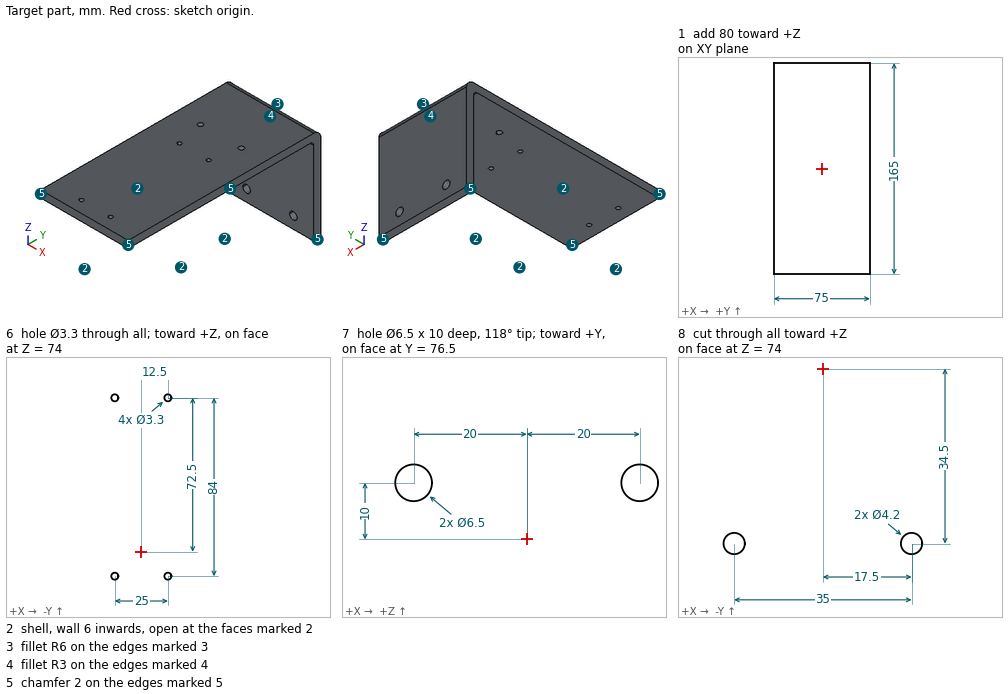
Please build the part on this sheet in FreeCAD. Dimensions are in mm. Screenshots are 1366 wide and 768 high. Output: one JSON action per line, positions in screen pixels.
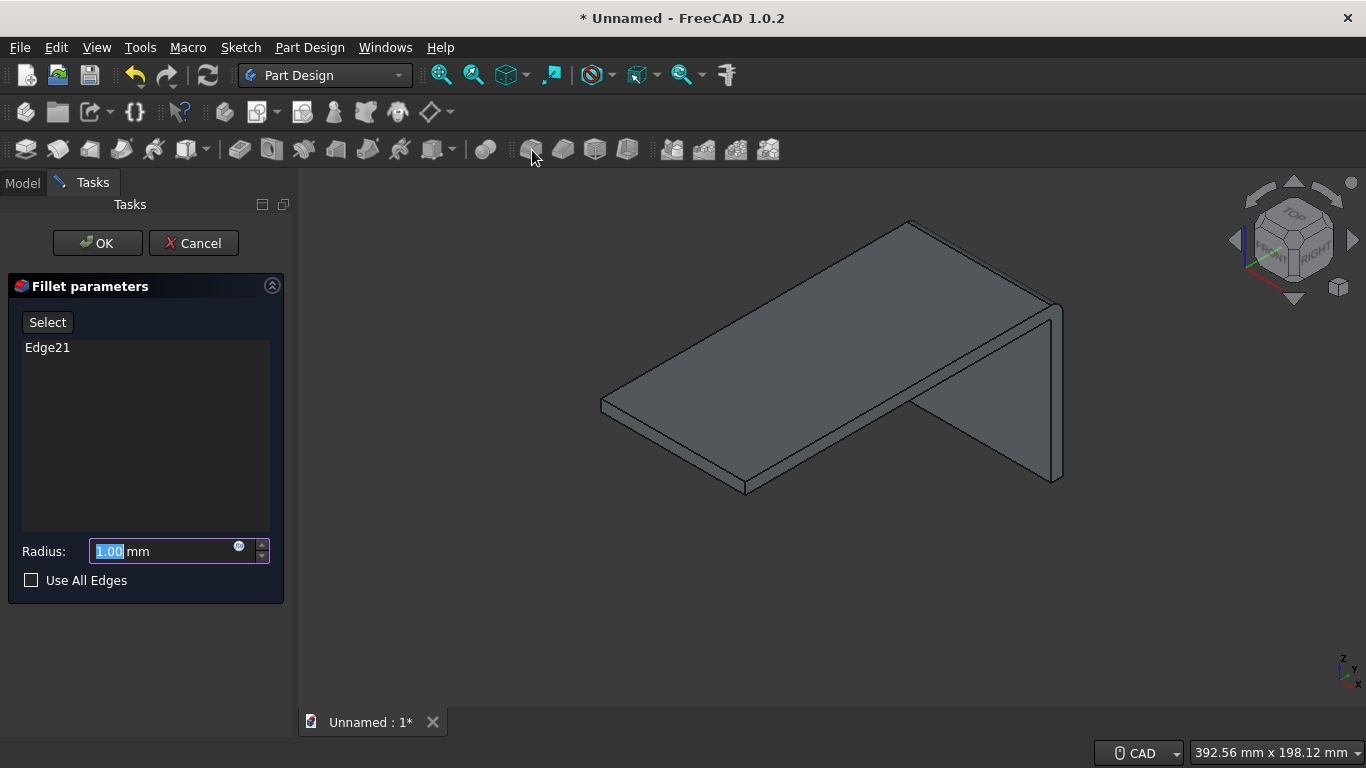
{"action": "type", "text": "3"}
{"action": "key", "text": "Tab"}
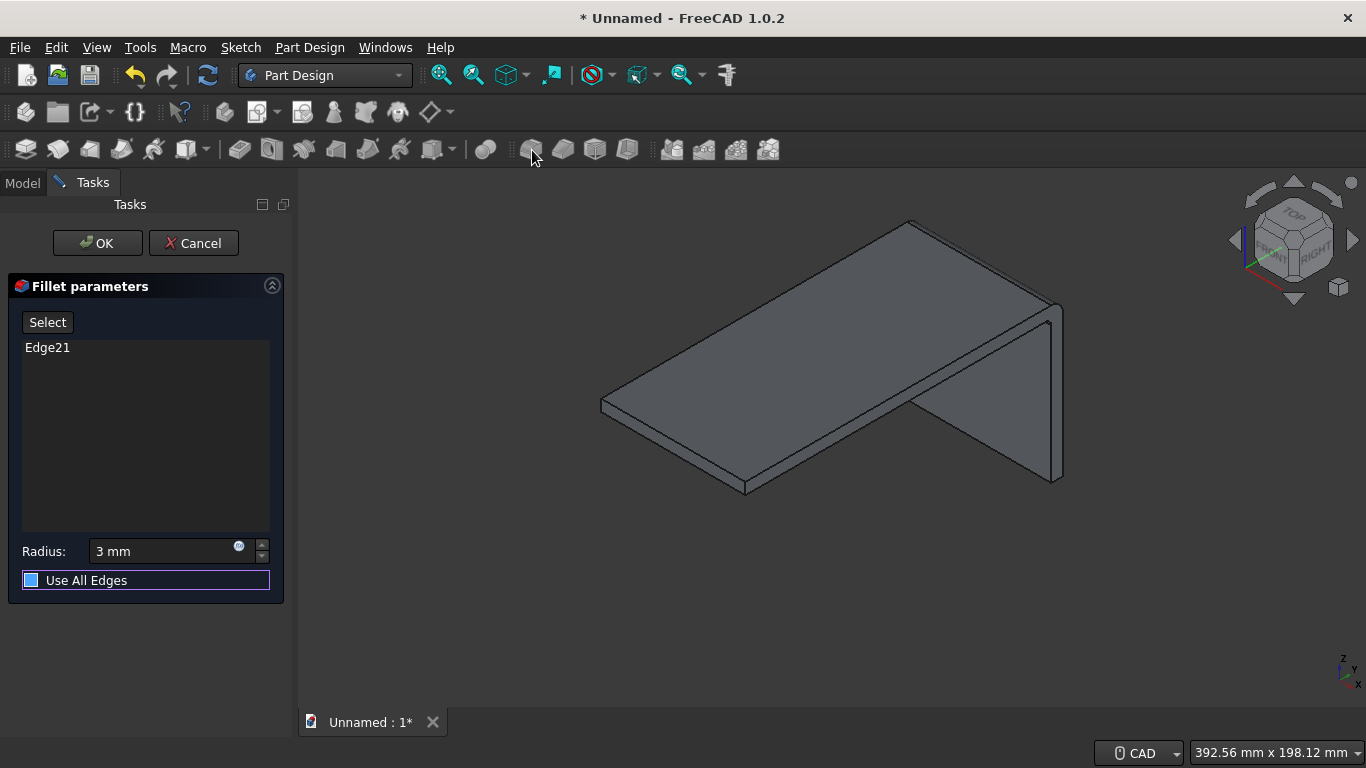
{"action": "left_click", "coordinate": [98, 243]}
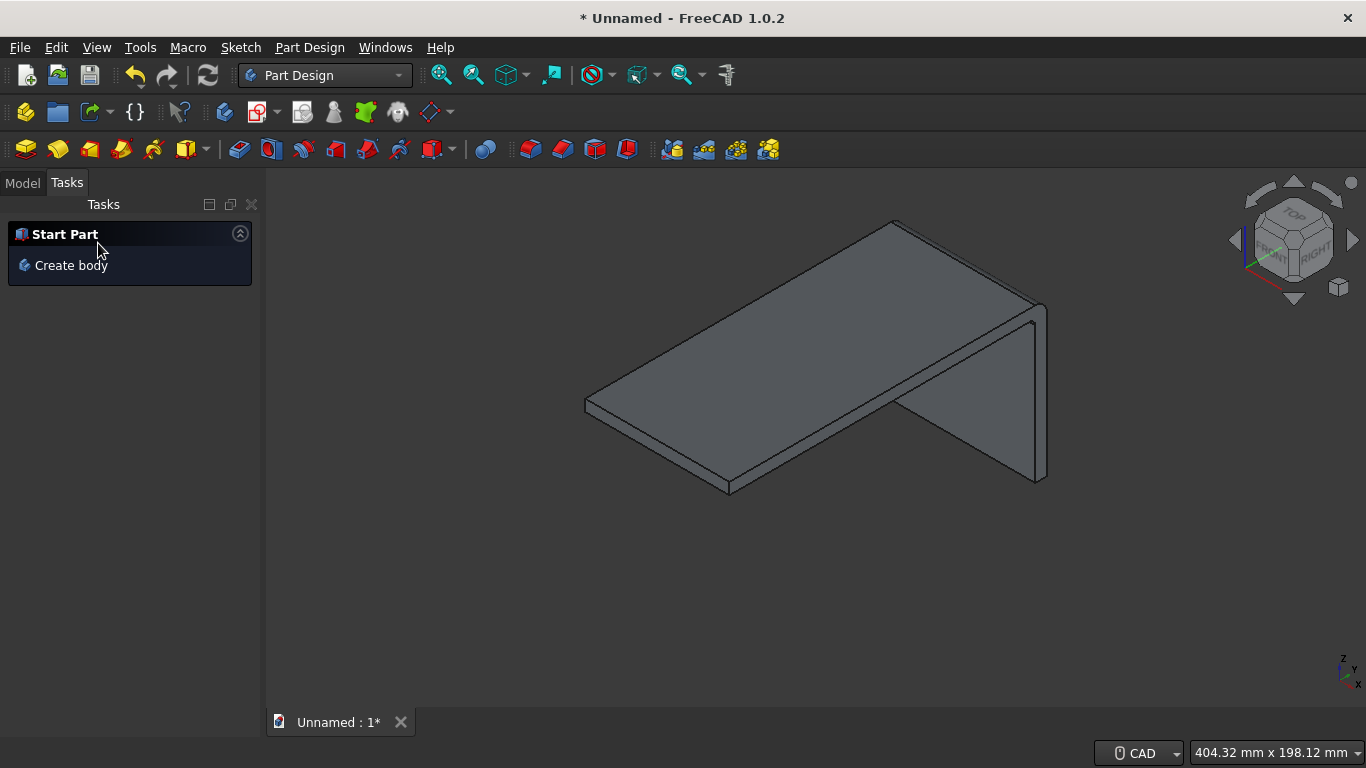
{"action": "left_click", "coordinate": [729, 488]}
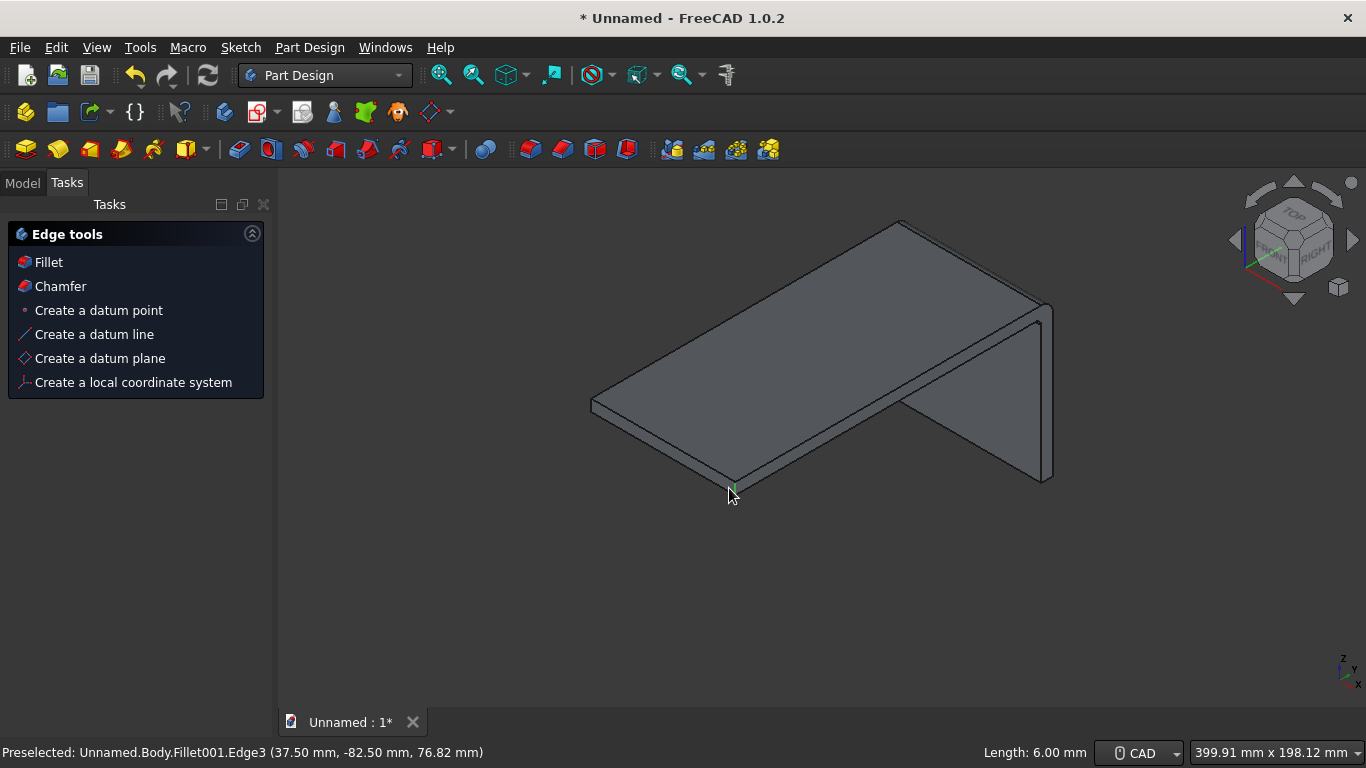
{"action": "scroll", "coordinate": [903, 395], "scroll_direction": "up", "scroll_amount": 5}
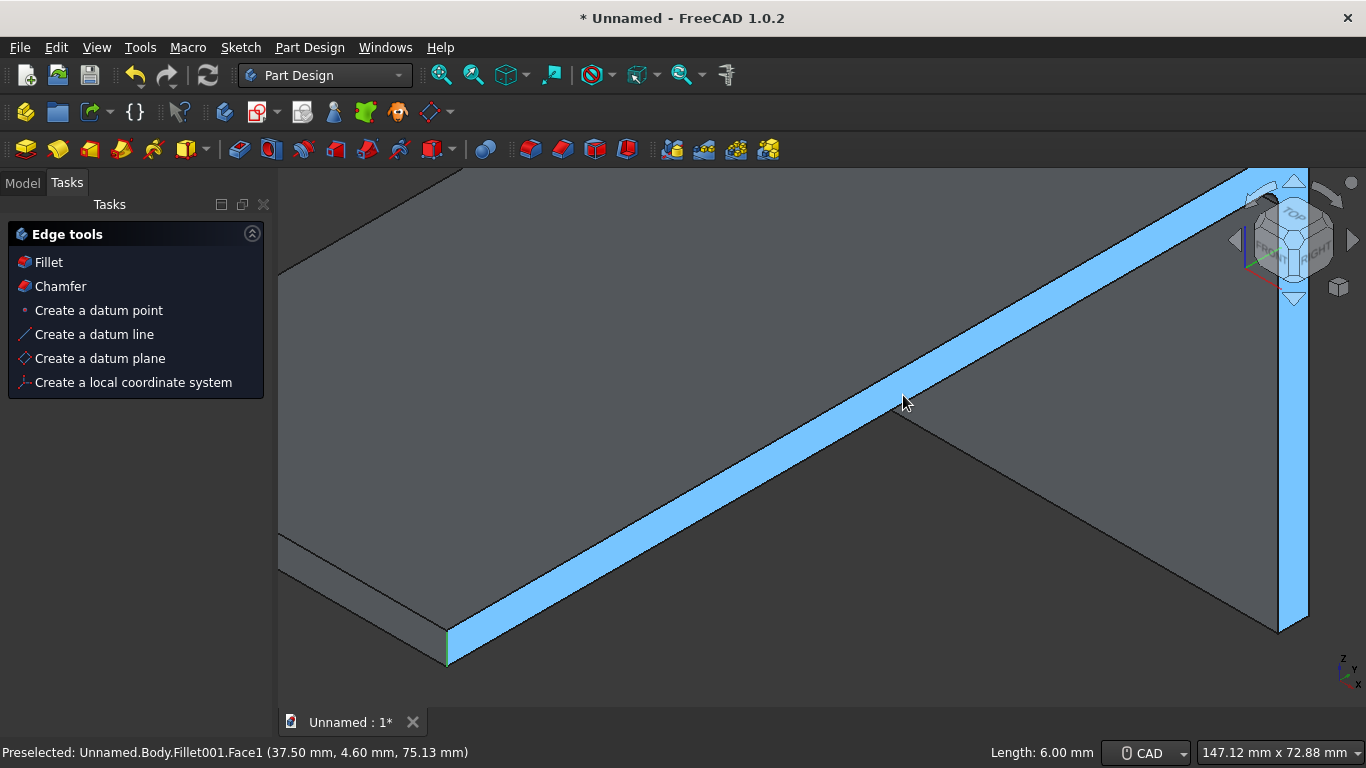
{"action": "left_click", "coordinate": [442, 76]}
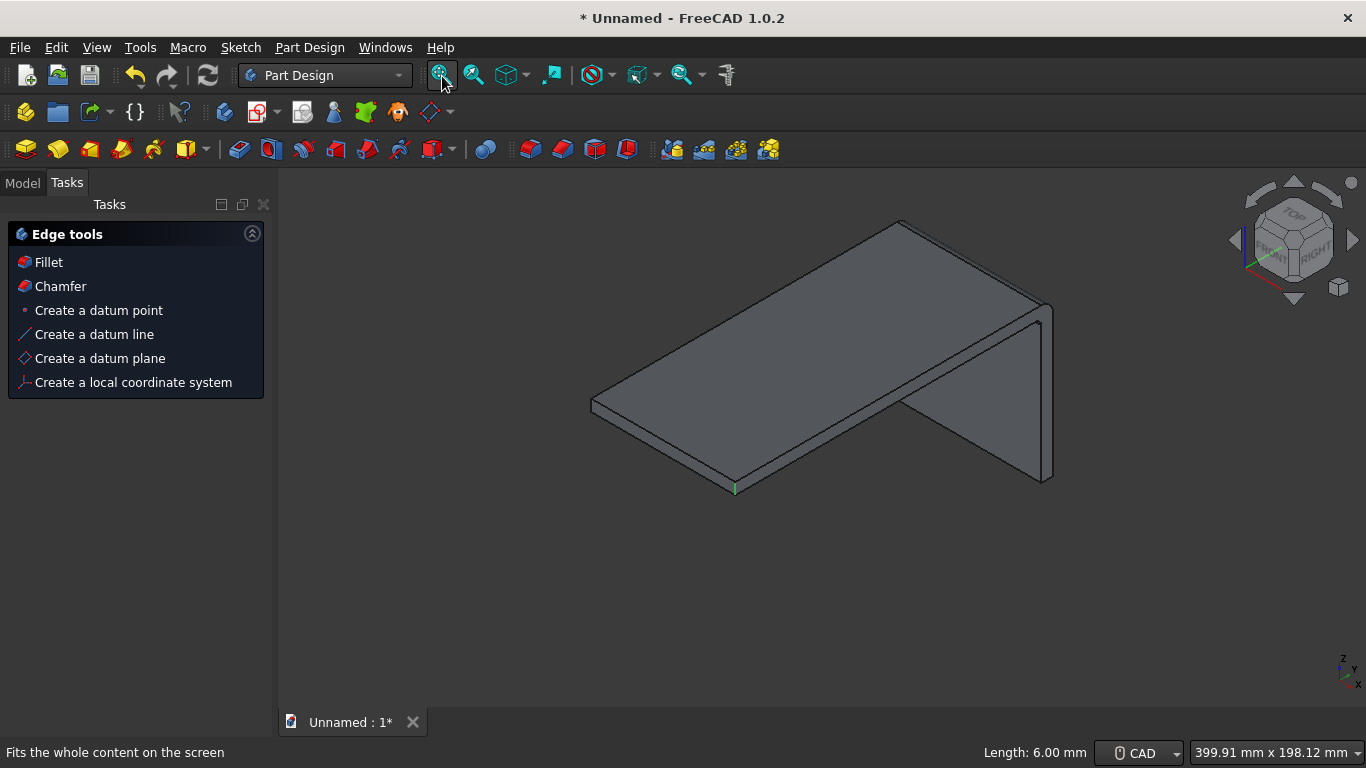
{"action": "key", "text": "2"}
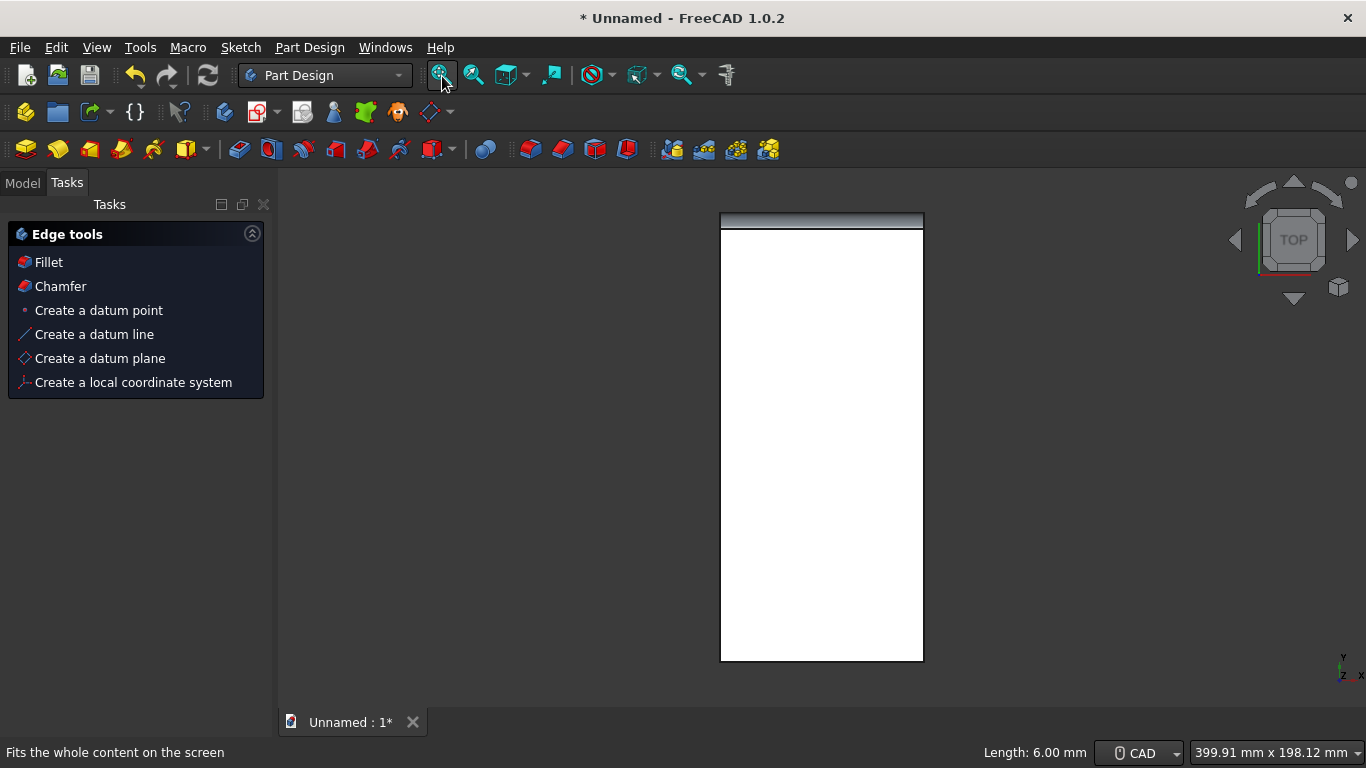
{"action": "scroll", "coordinate": [720, 220], "scroll_direction": "up", "scroll_amount": 5}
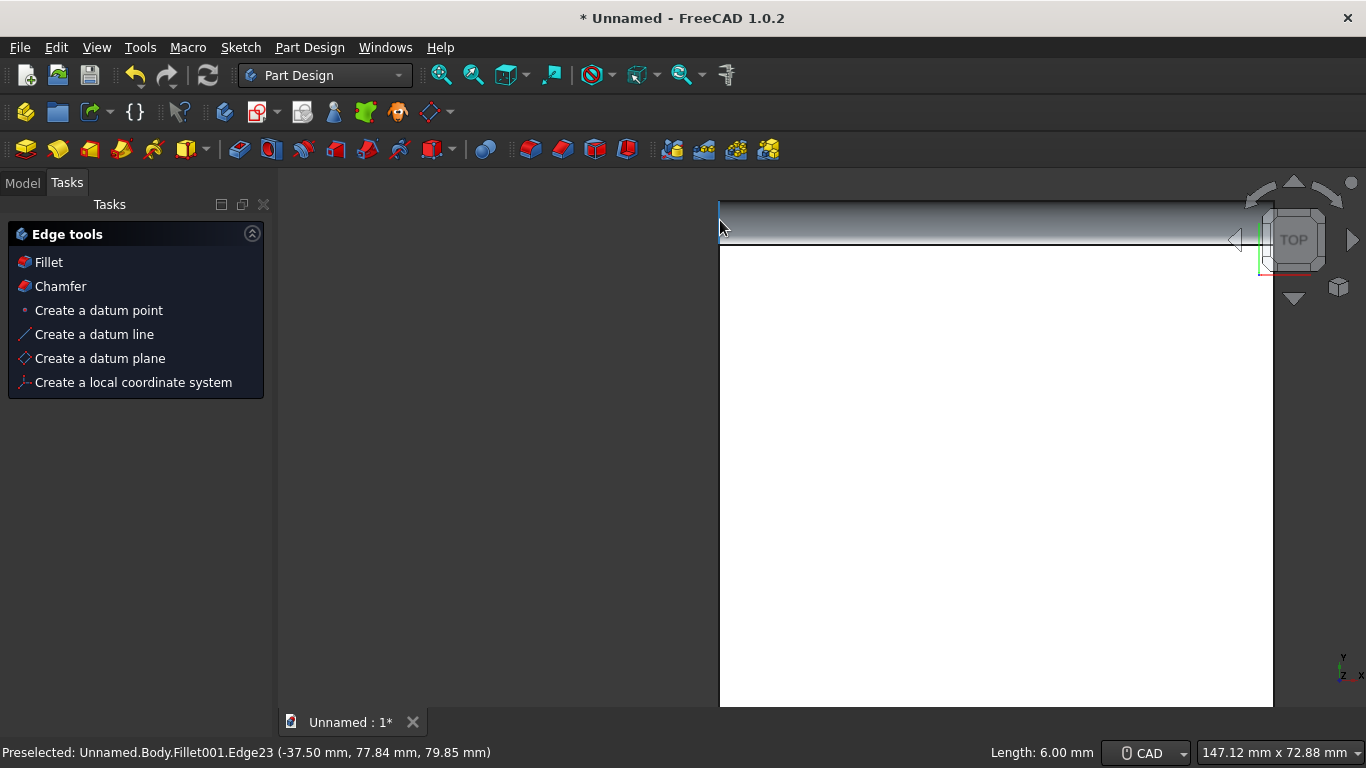
{"action": "left_click", "coordinate": [442, 76]}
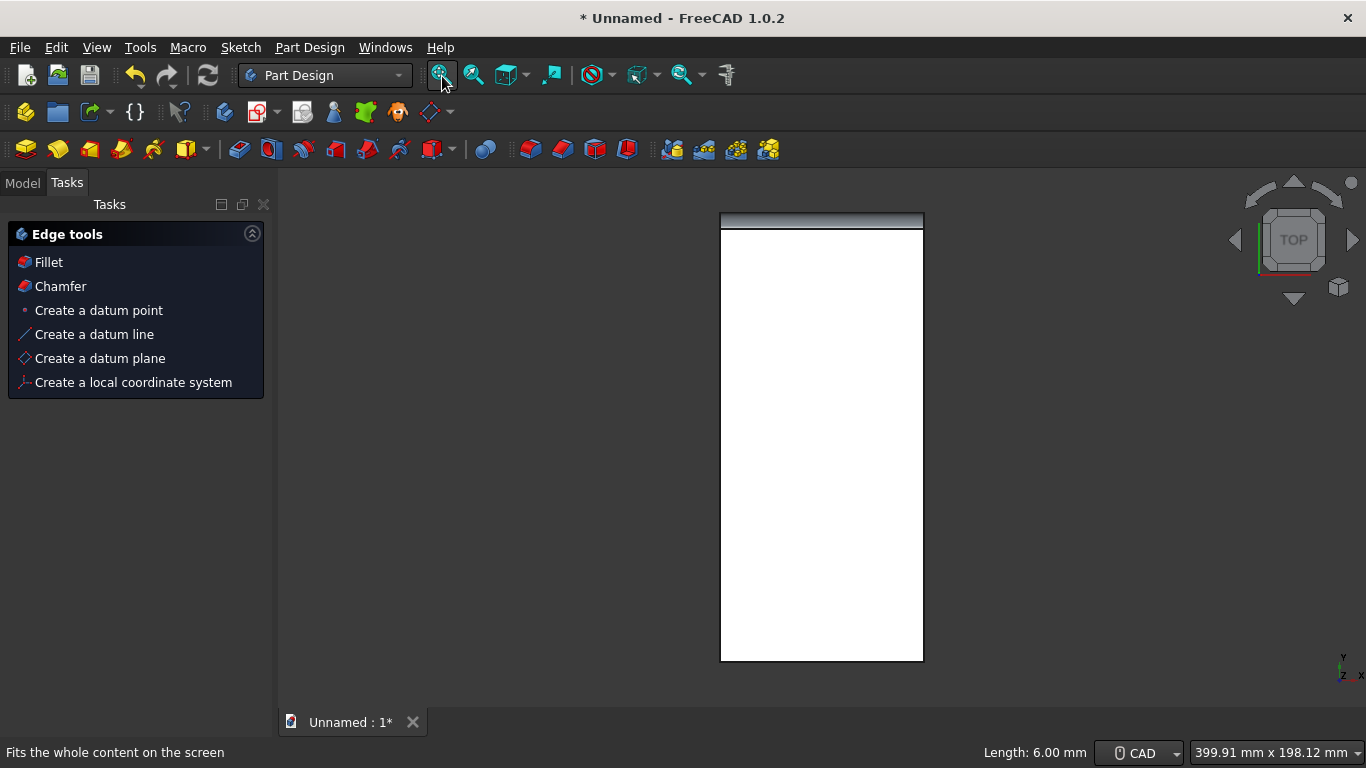
{"action": "key", "text": "0"}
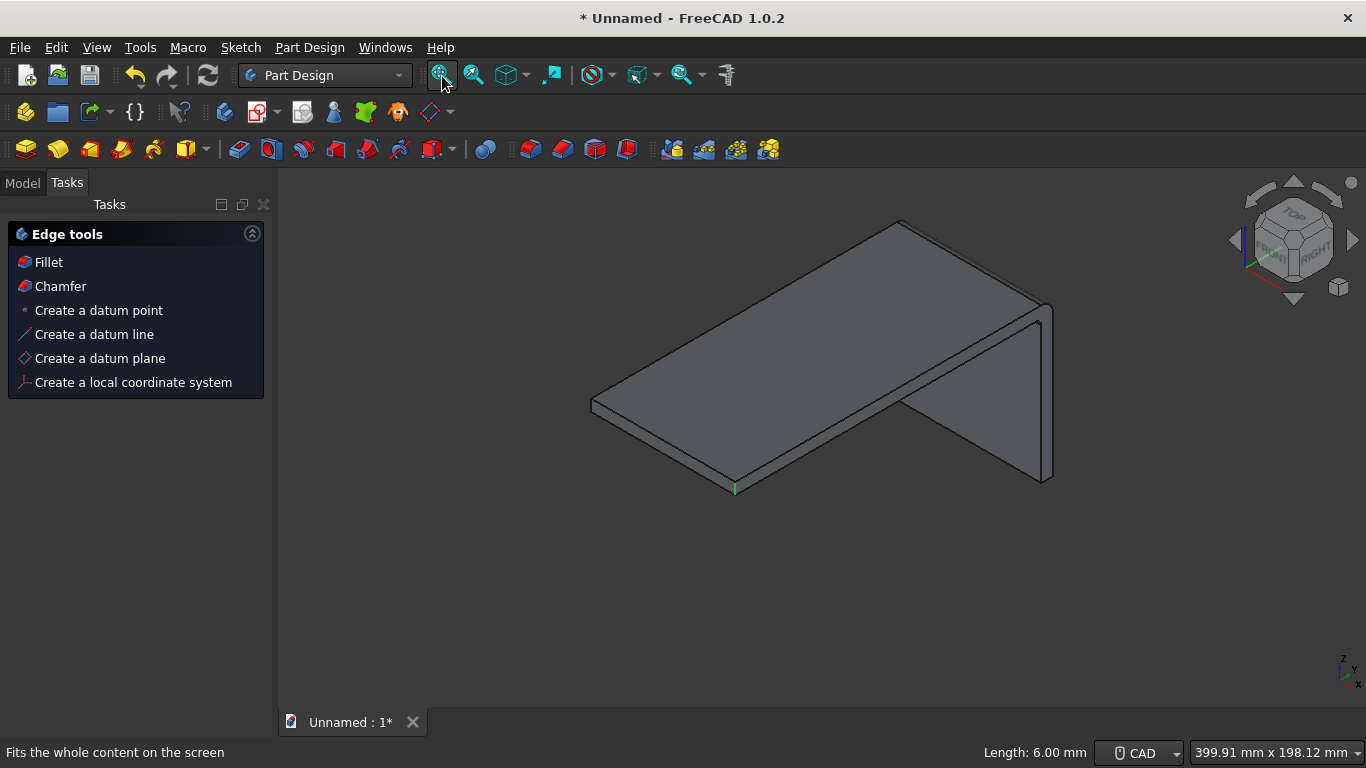
{"action": "scroll", "coordinate": [903, 395], "scroll_direction": "up", "scroll_amount": 5}